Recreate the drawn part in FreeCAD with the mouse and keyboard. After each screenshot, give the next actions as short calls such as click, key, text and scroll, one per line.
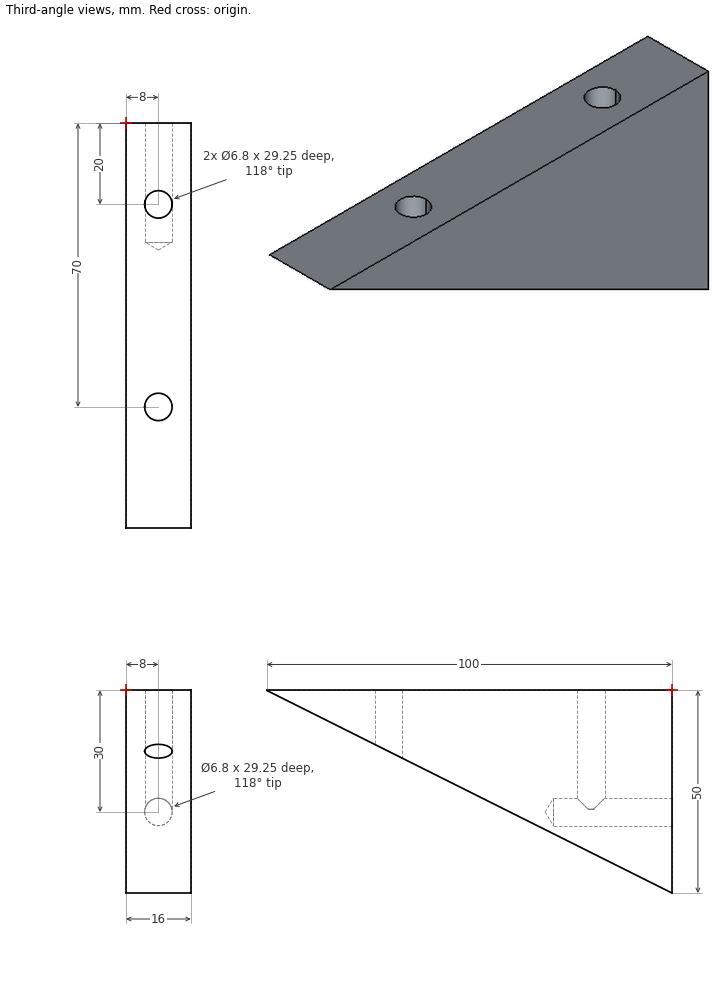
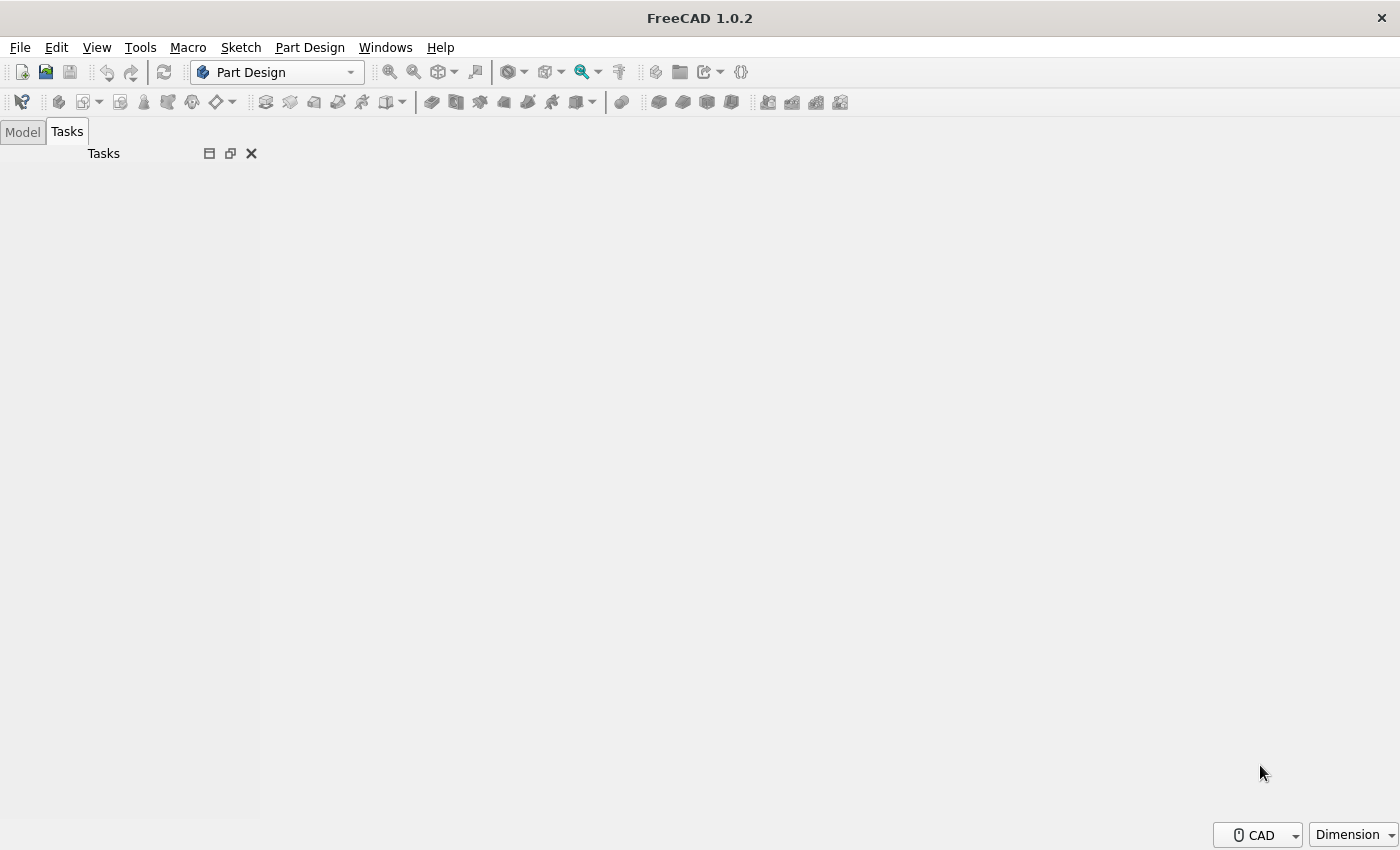
key(ctrl+n)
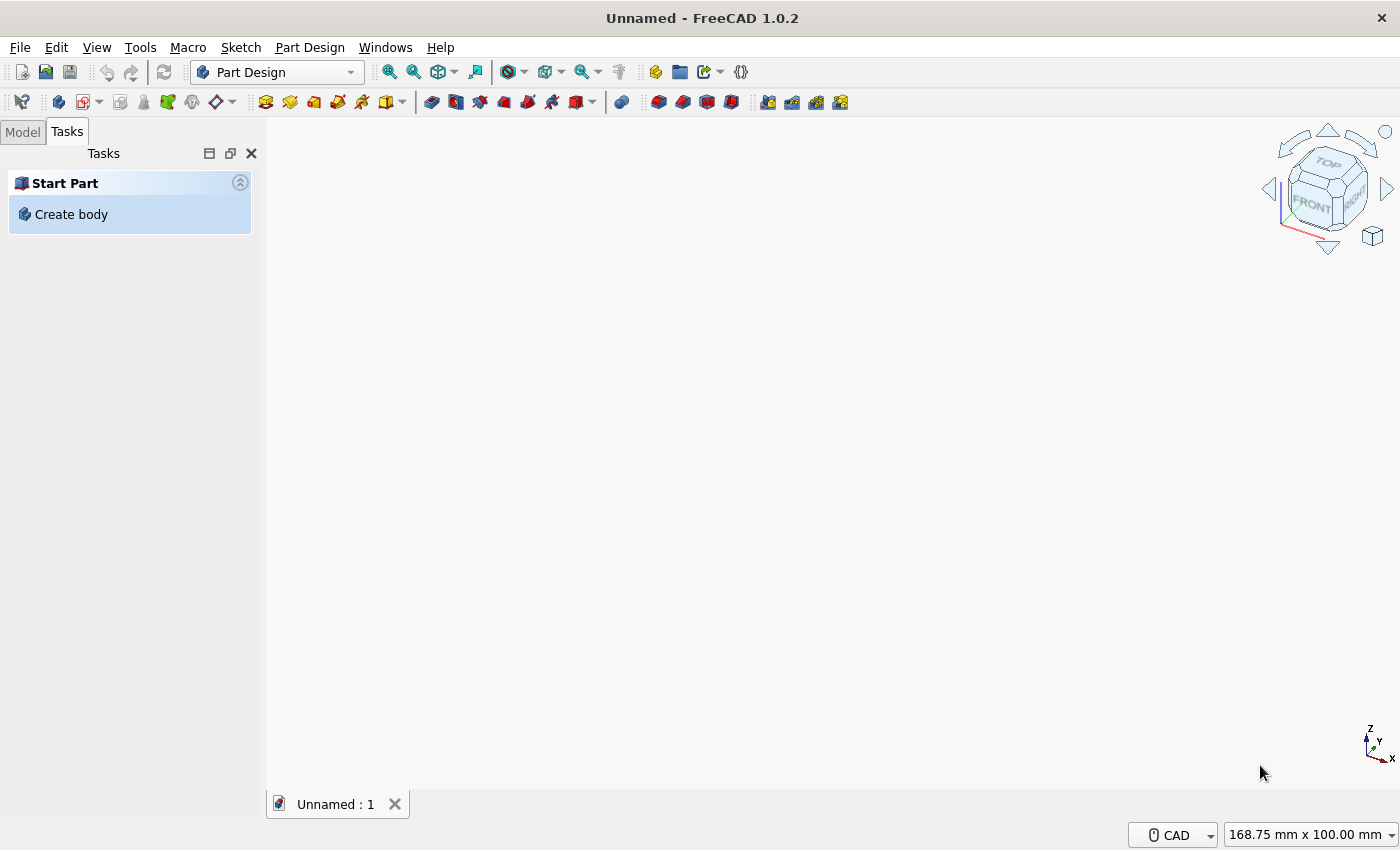
click(84, 102)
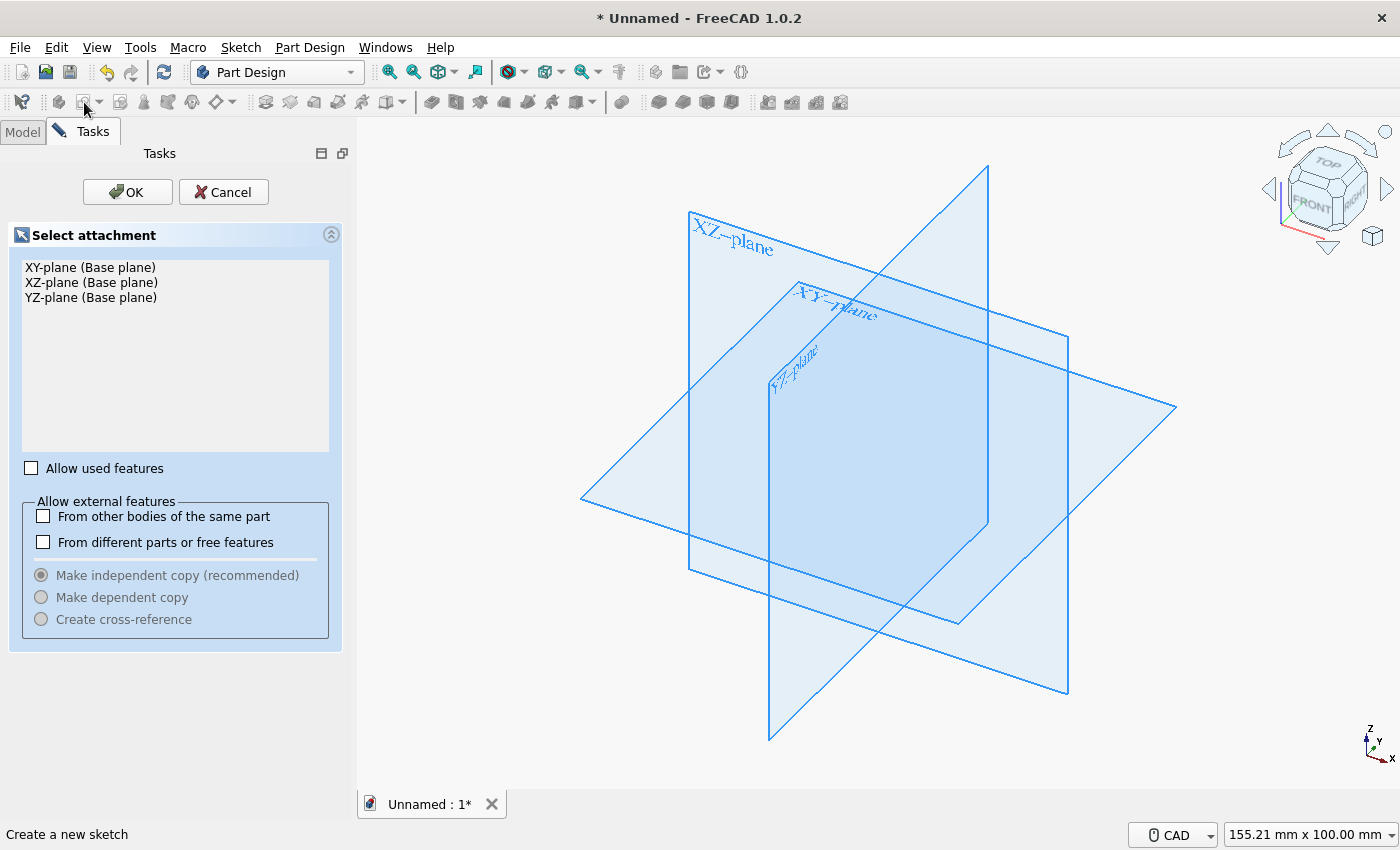
click(82, 298)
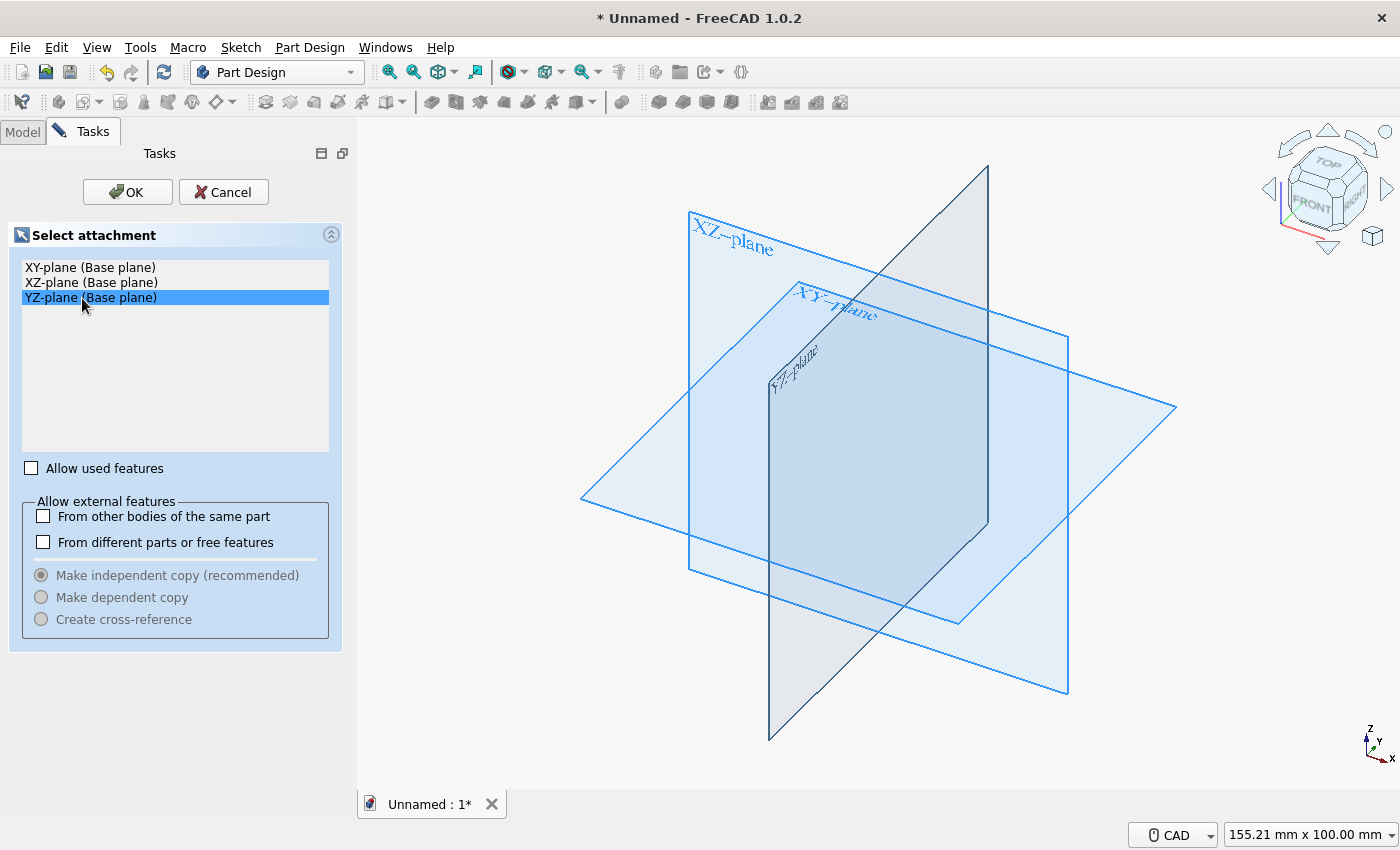
click(128, 192)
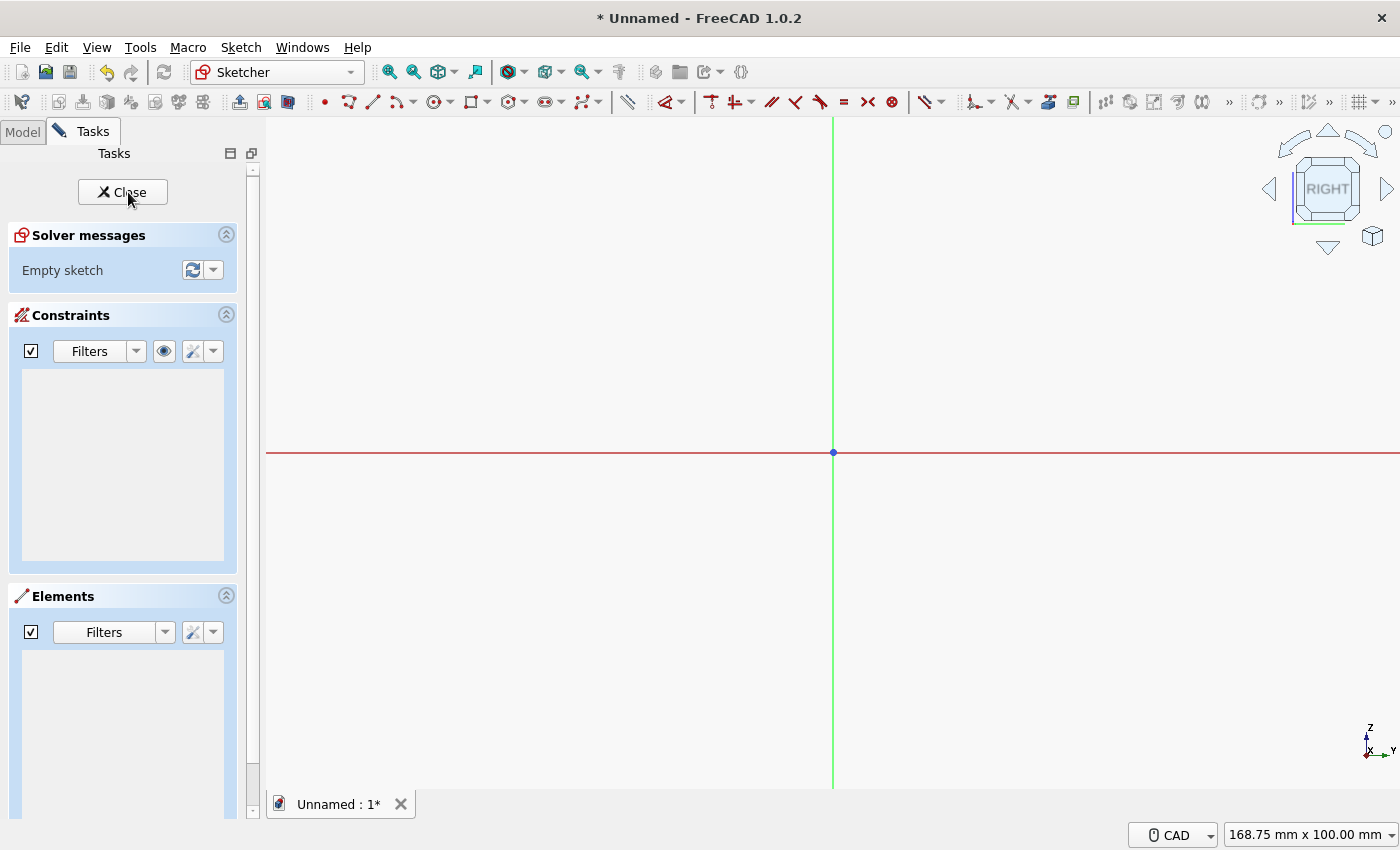
scroll(1235, 145, down, 1)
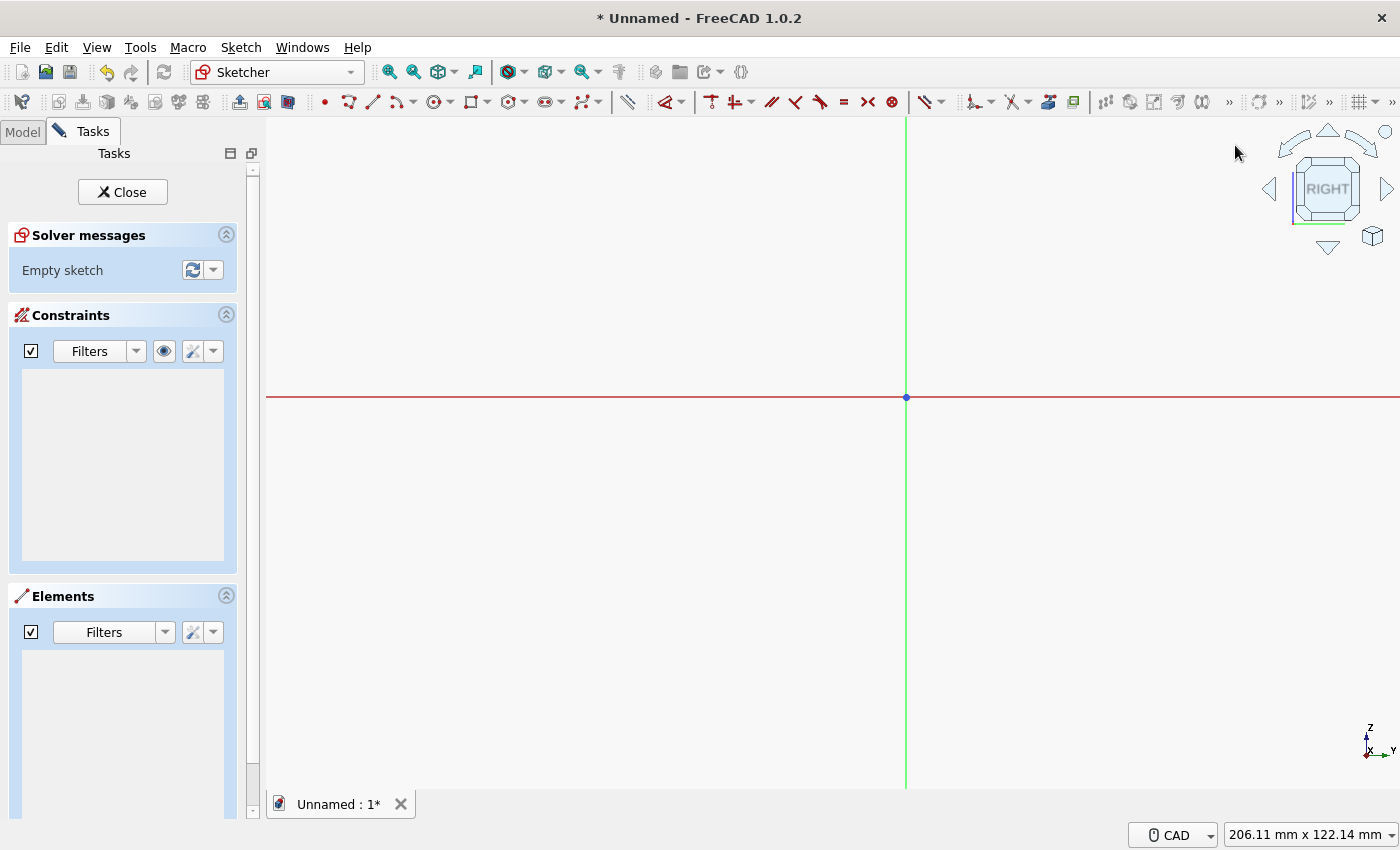
key(g)
key(m)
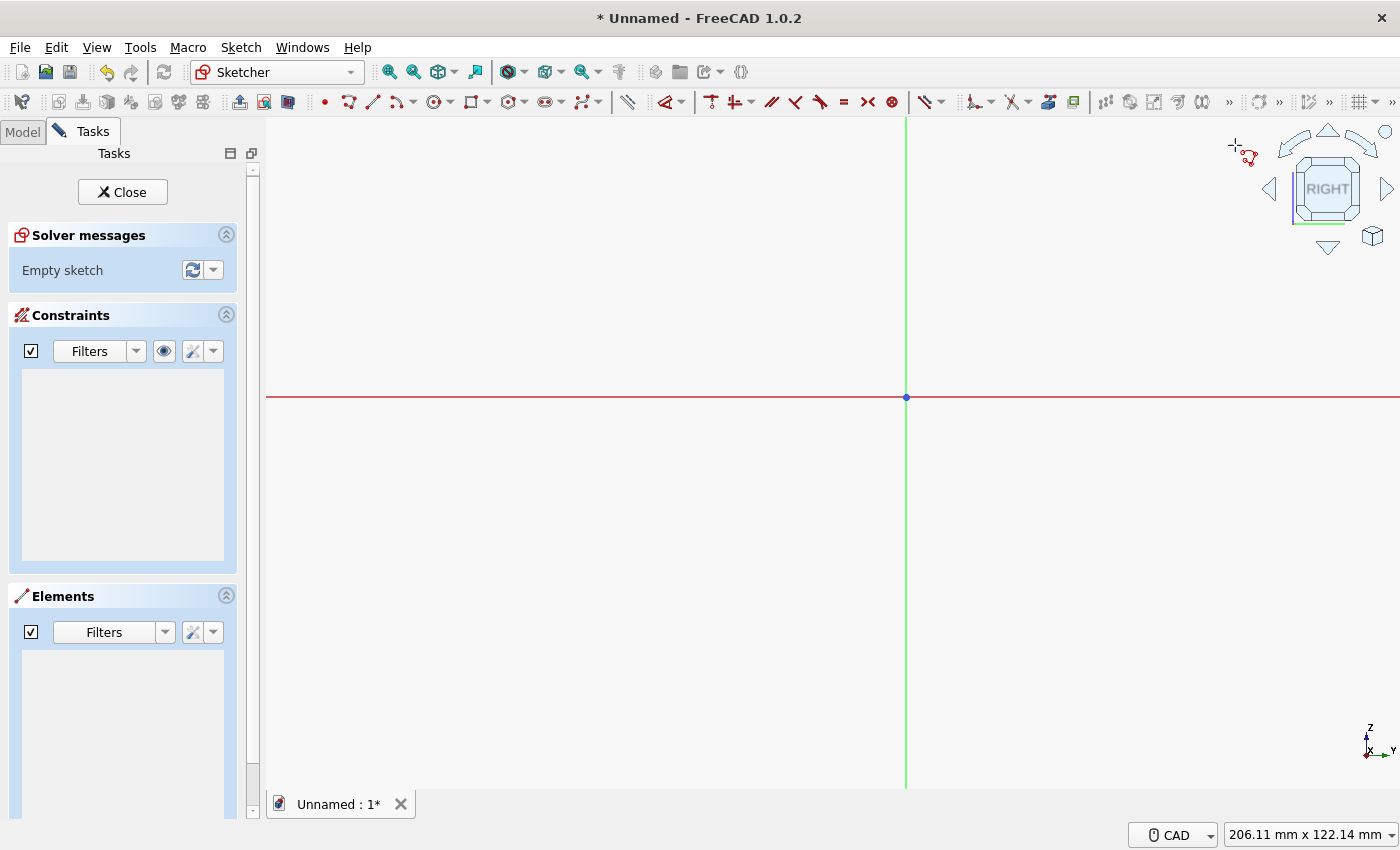
click(906, 397)
click(356, 406)
click(897, 672)
click(906, 397)
key(Escape)
key(Escape)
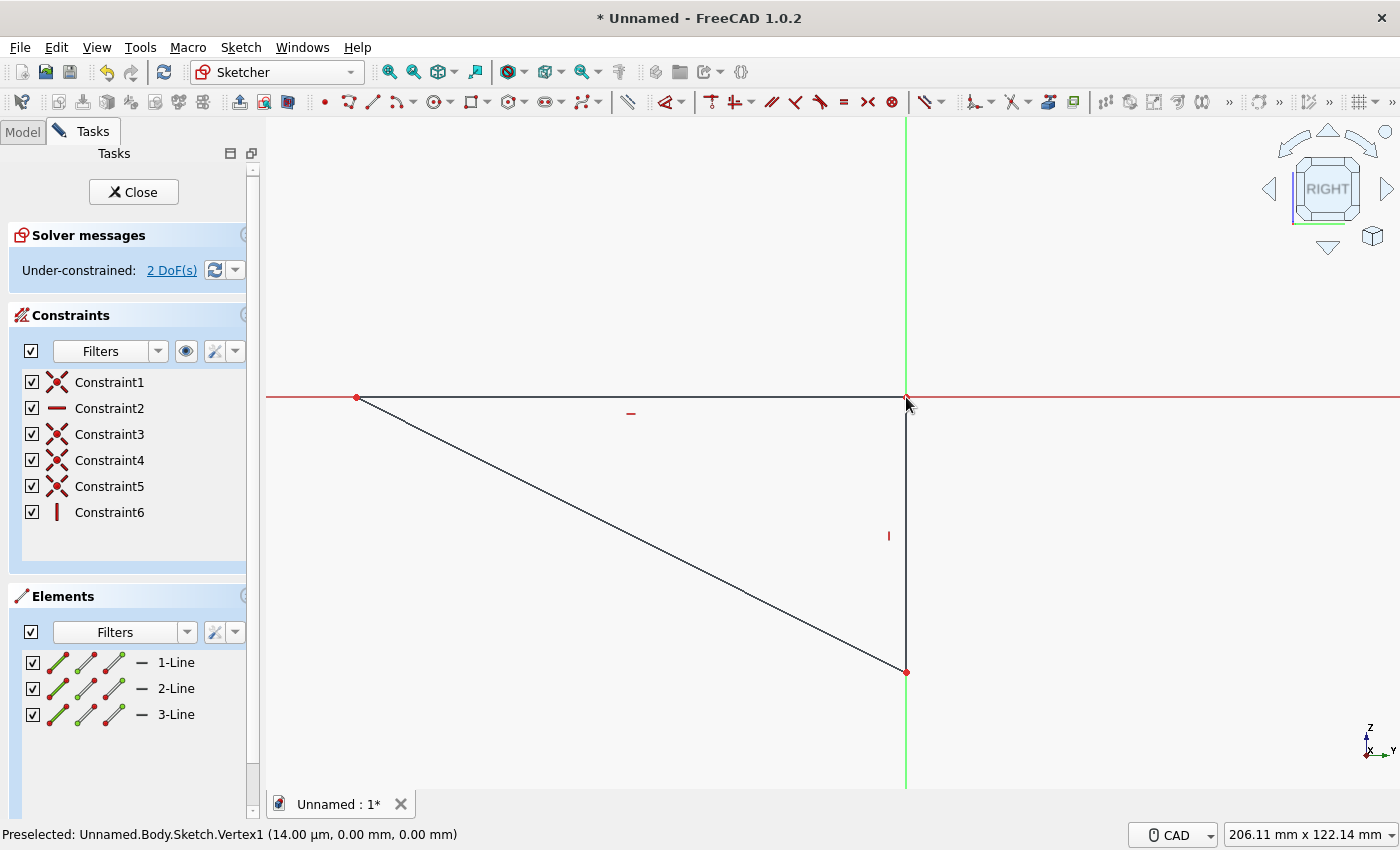
click(666, 102)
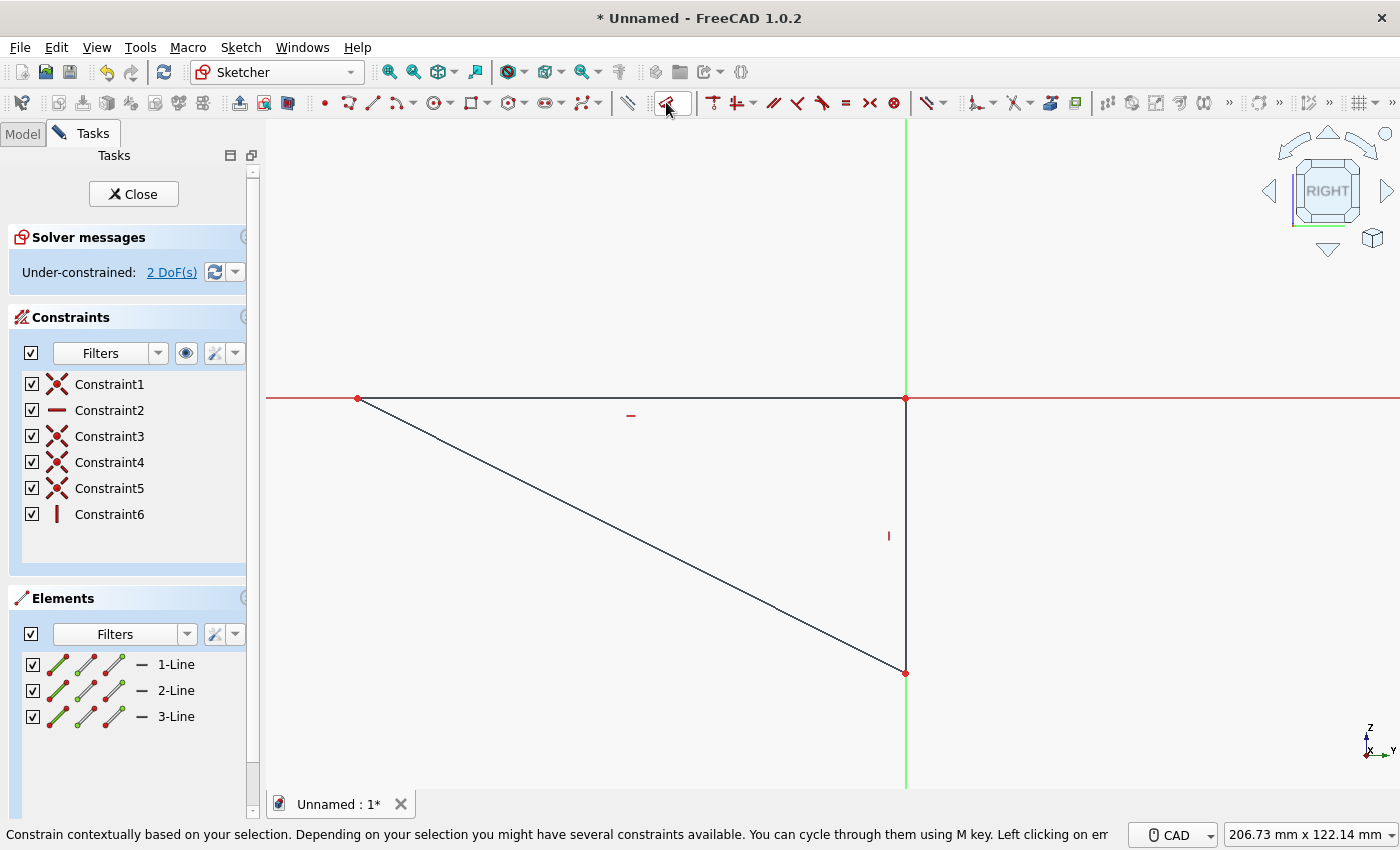
click(906, 591)
click(940, 536)